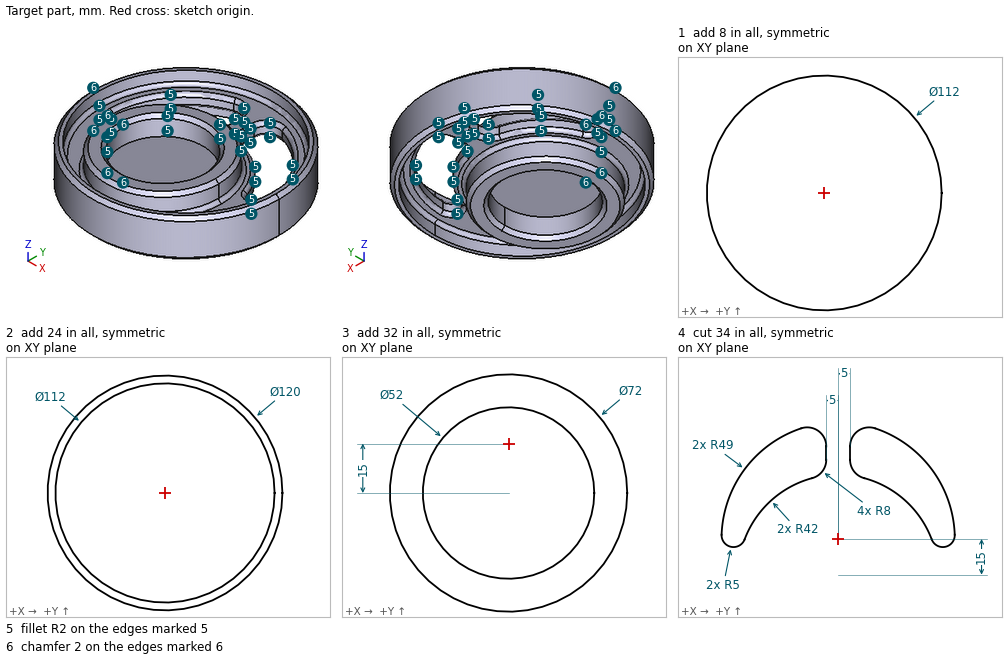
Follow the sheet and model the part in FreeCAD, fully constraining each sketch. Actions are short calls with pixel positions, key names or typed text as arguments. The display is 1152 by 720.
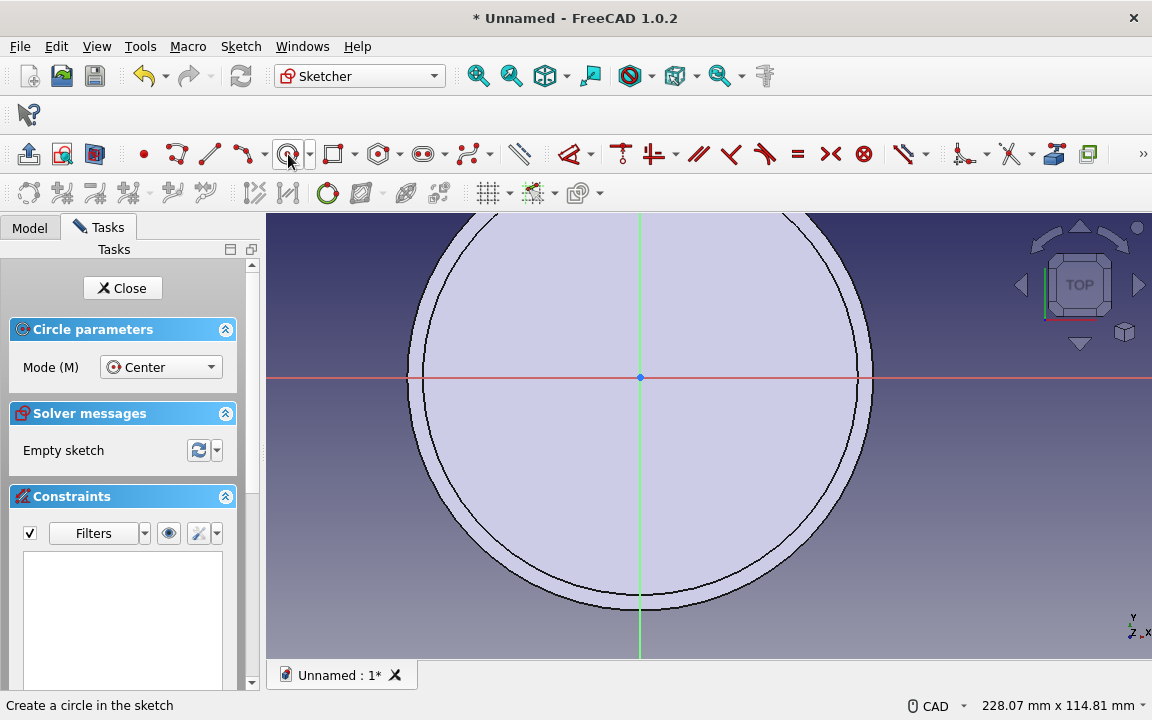
click(640, 436)
move(739, 337)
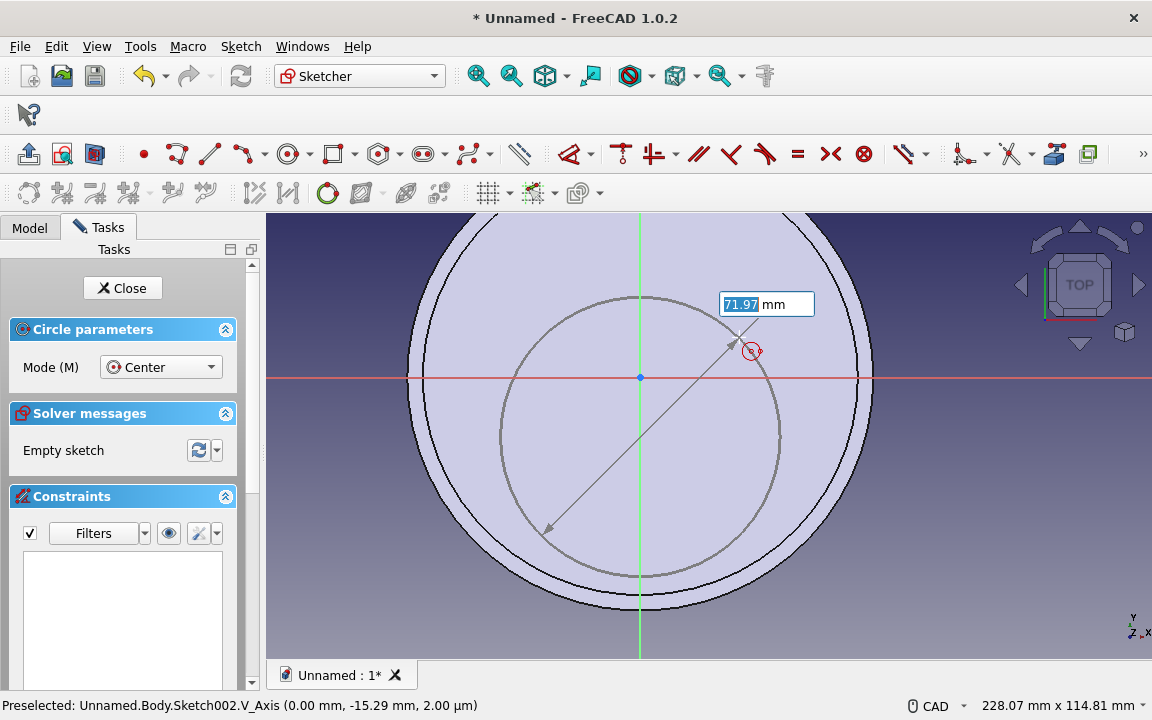
text(72)
key(Return)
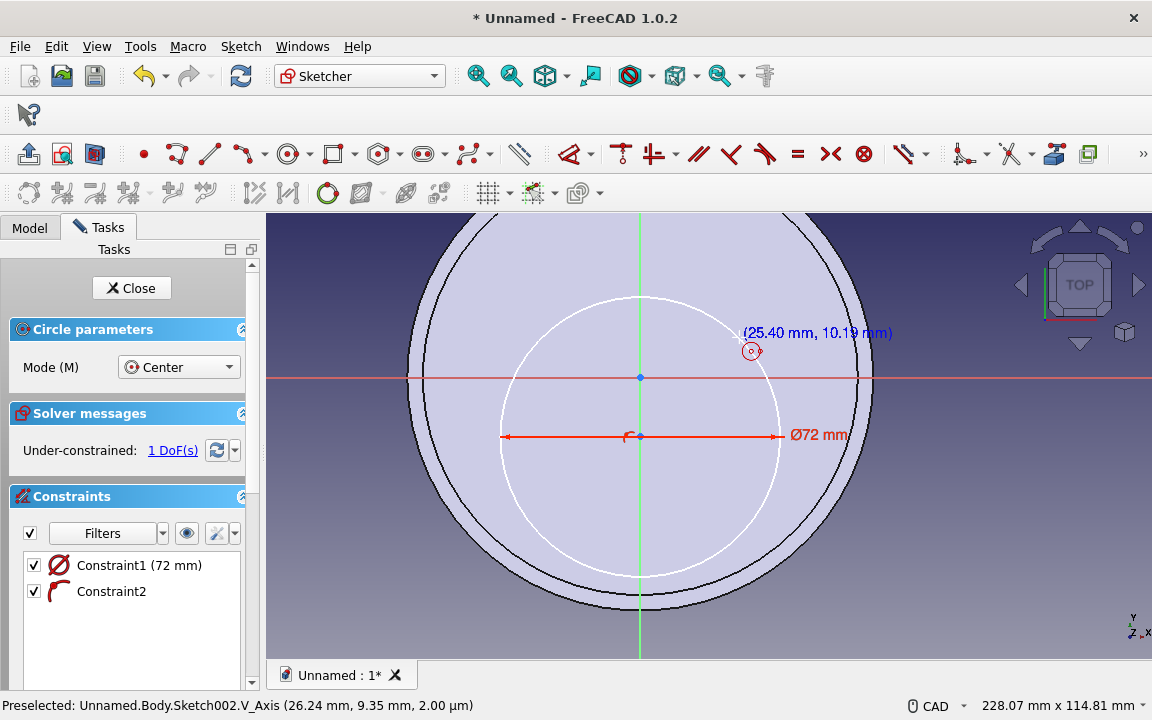
click(640, 437)
move(712, 507)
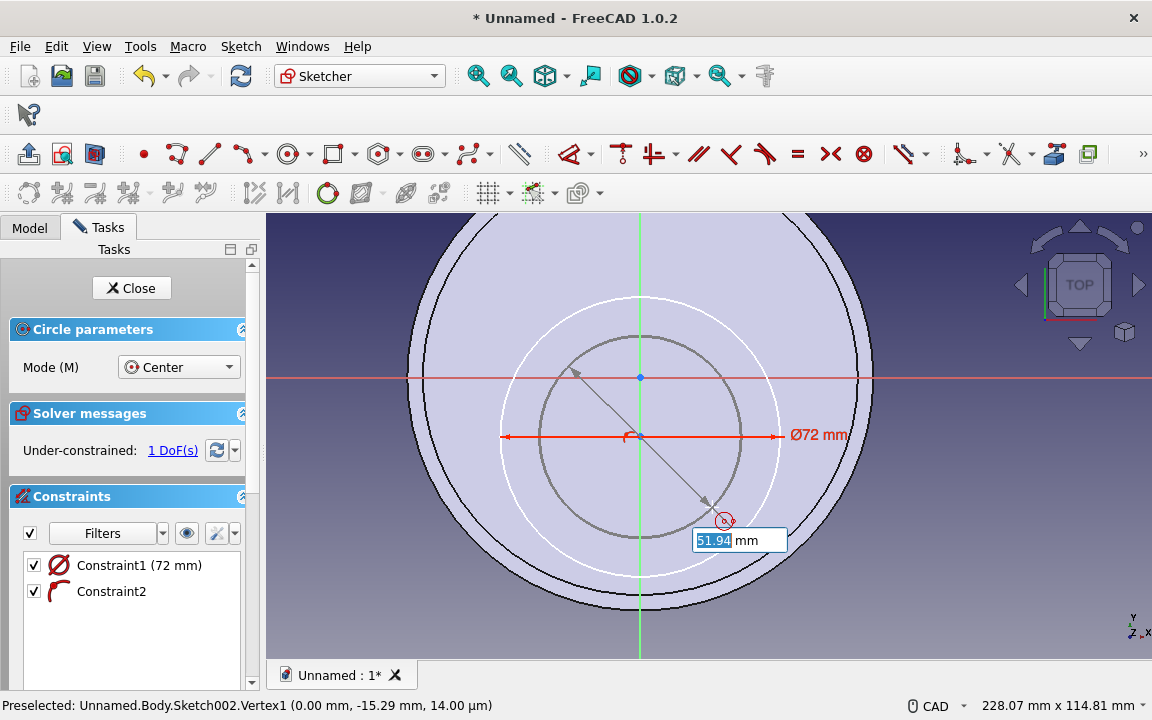
text(52)
key(Return)
key(Escape)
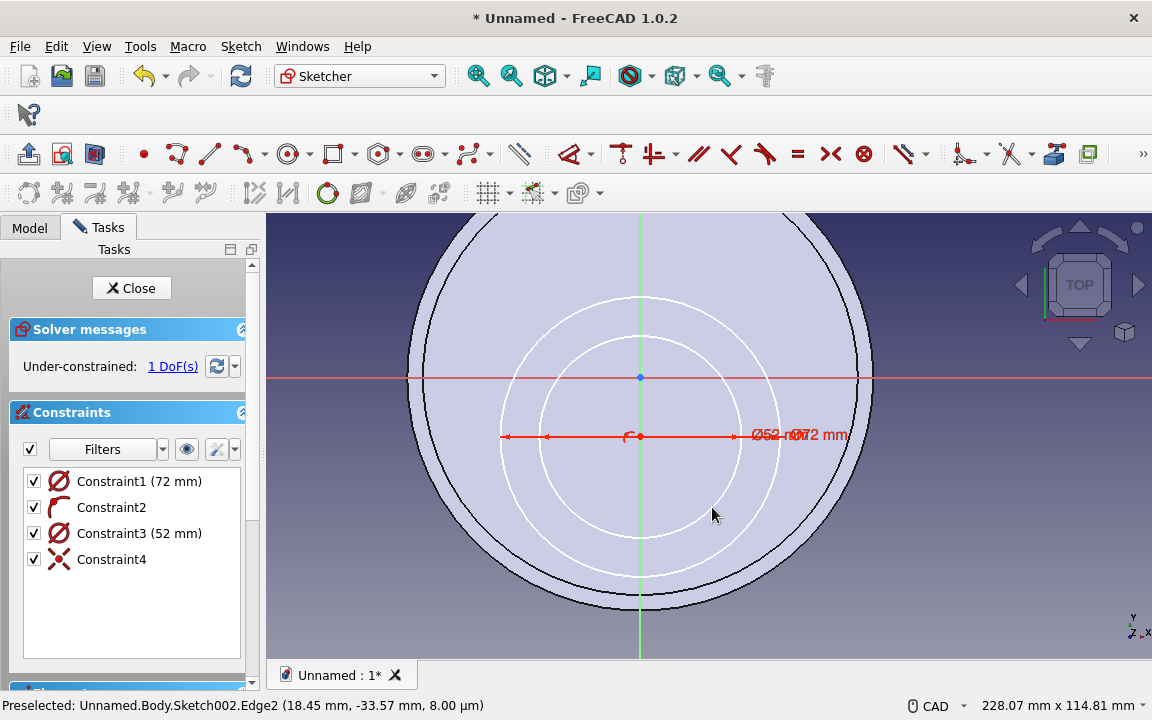
key(d)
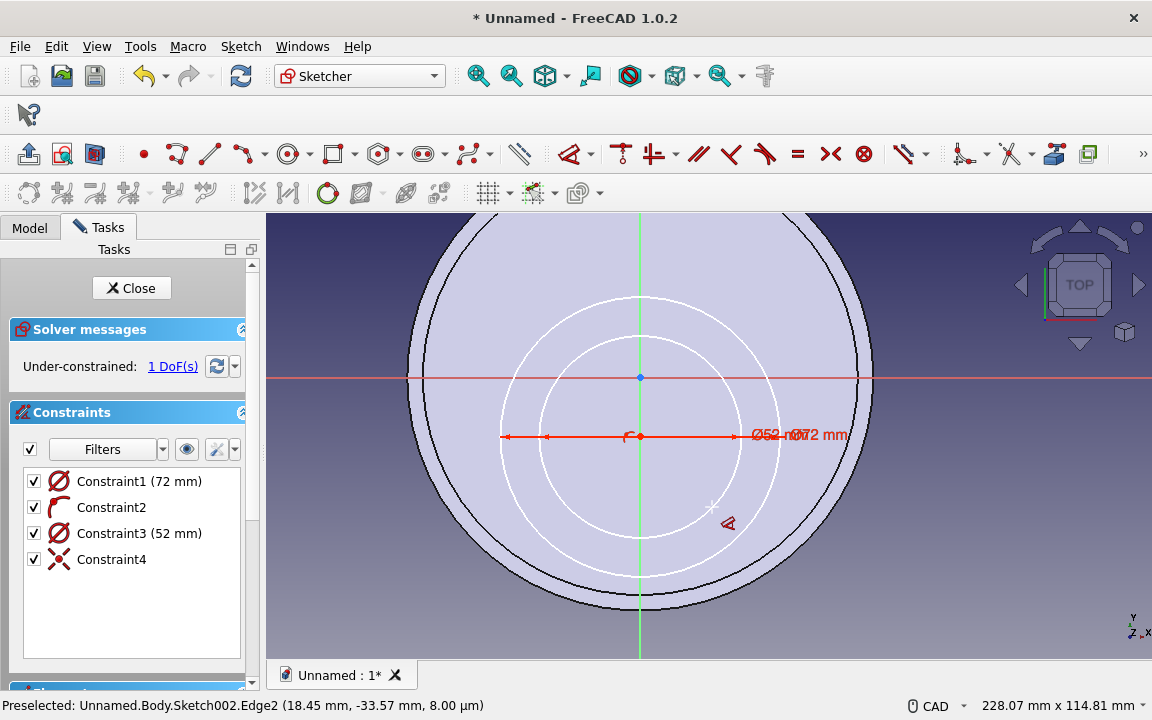
click(640, 437)
click(674, 407)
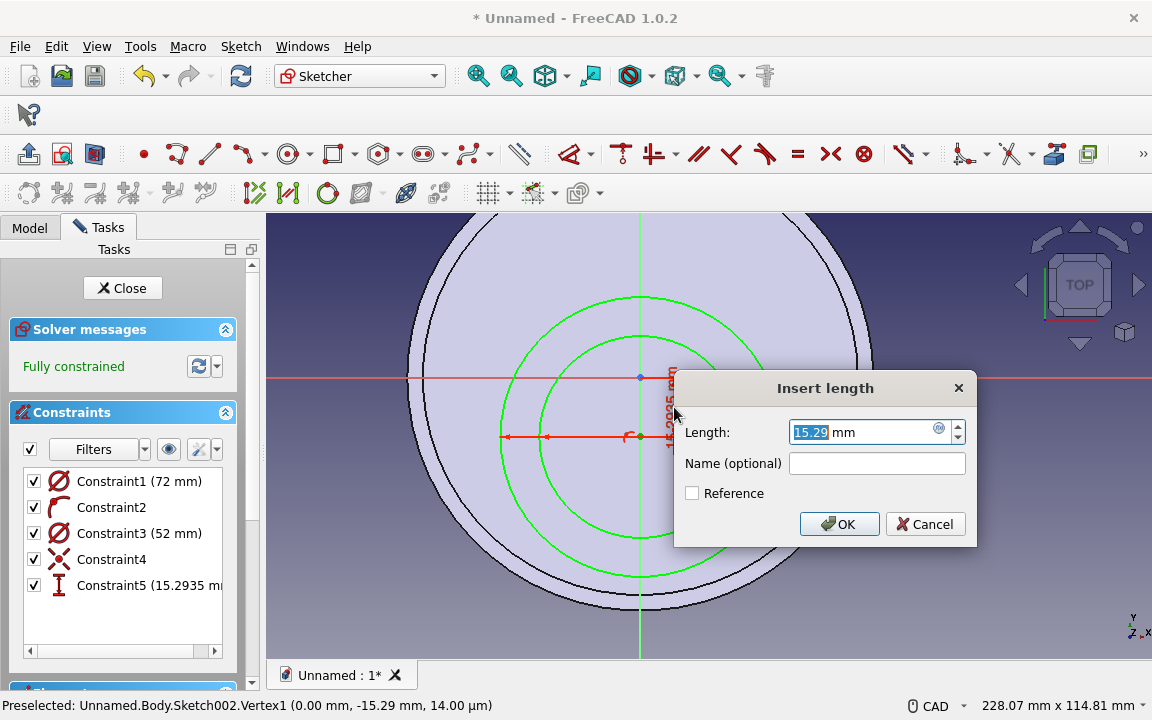
text(15)
key(Return)
key(Escape)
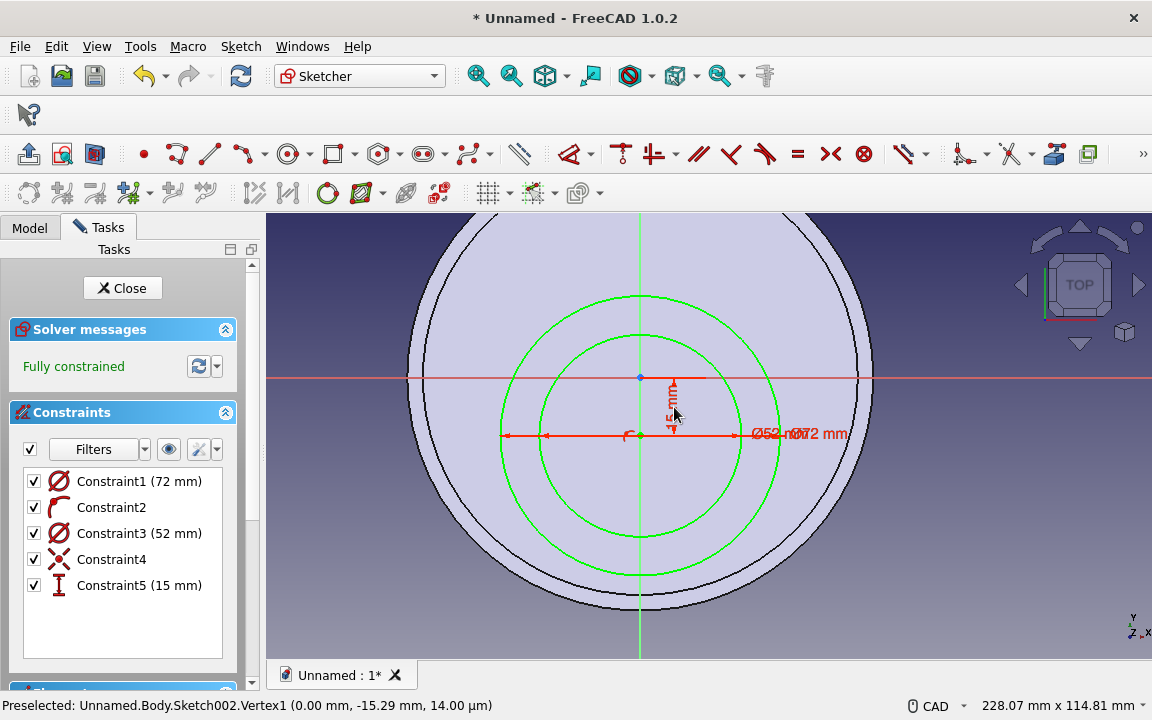
click(123, 288)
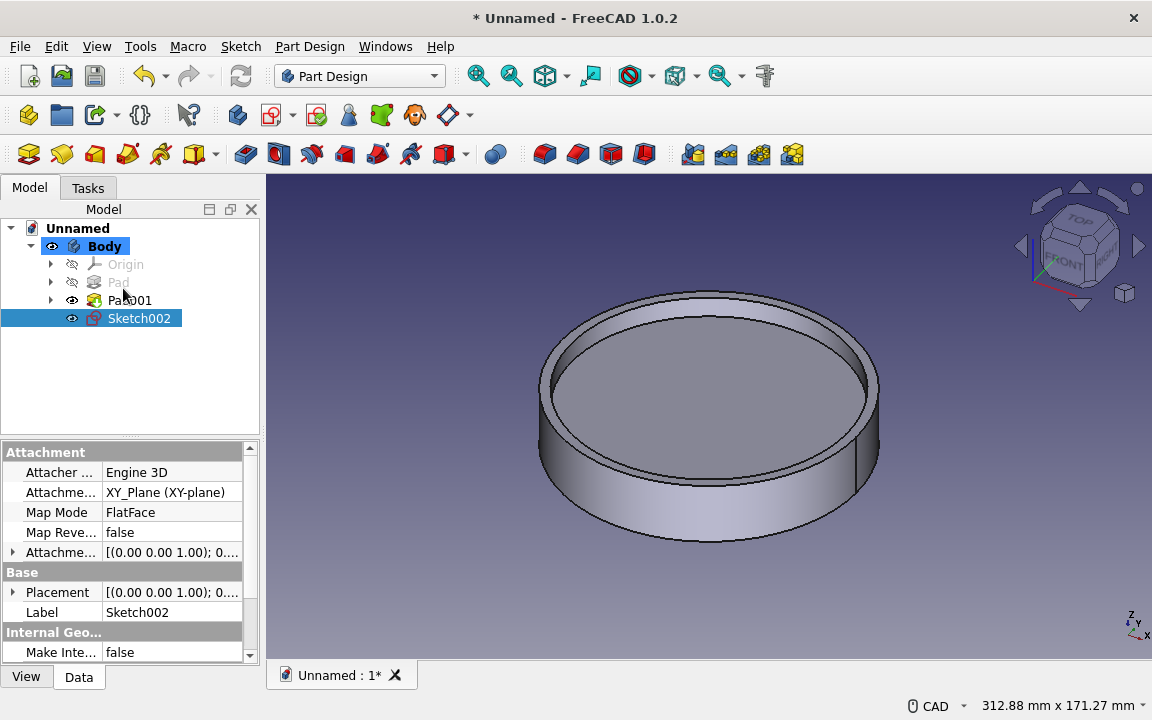
click(29, 154)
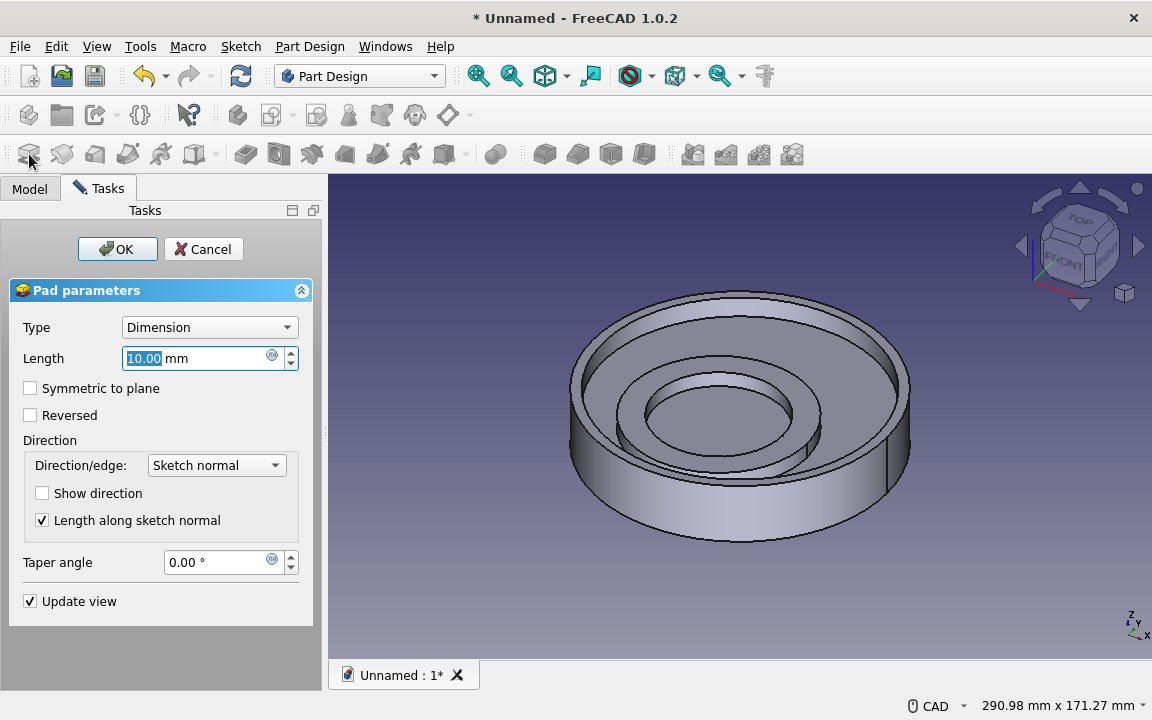
text(32)
key(Tab)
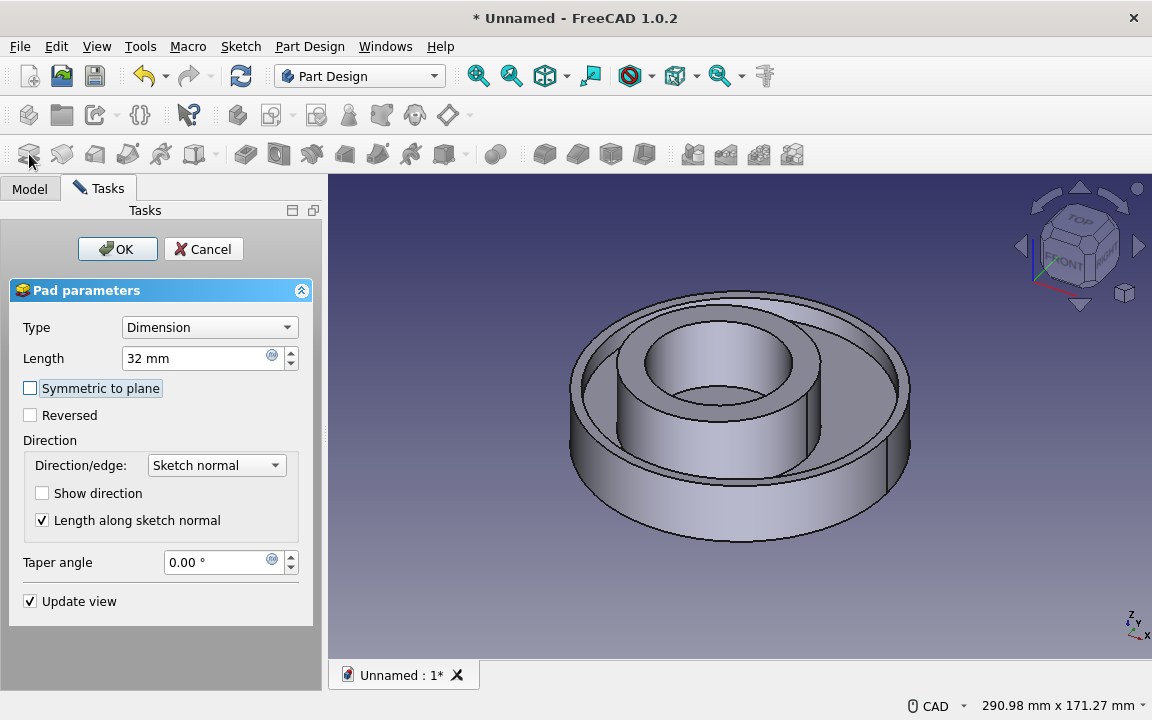
click(31, 388)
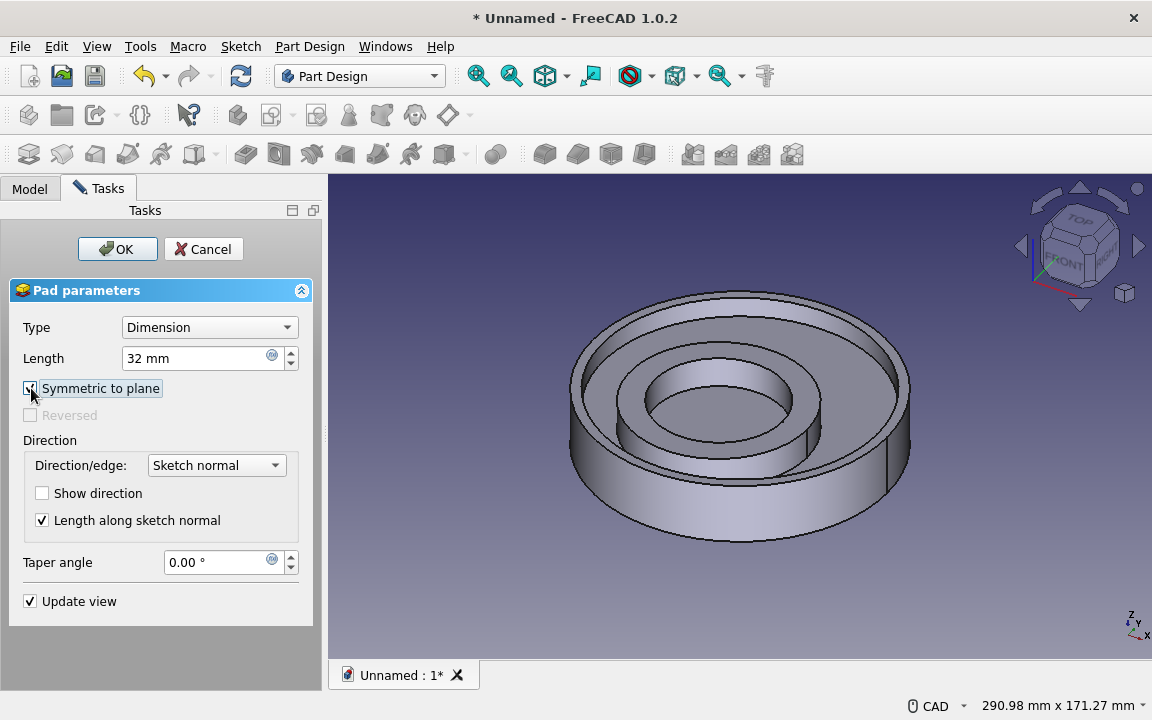
click(118, 249)